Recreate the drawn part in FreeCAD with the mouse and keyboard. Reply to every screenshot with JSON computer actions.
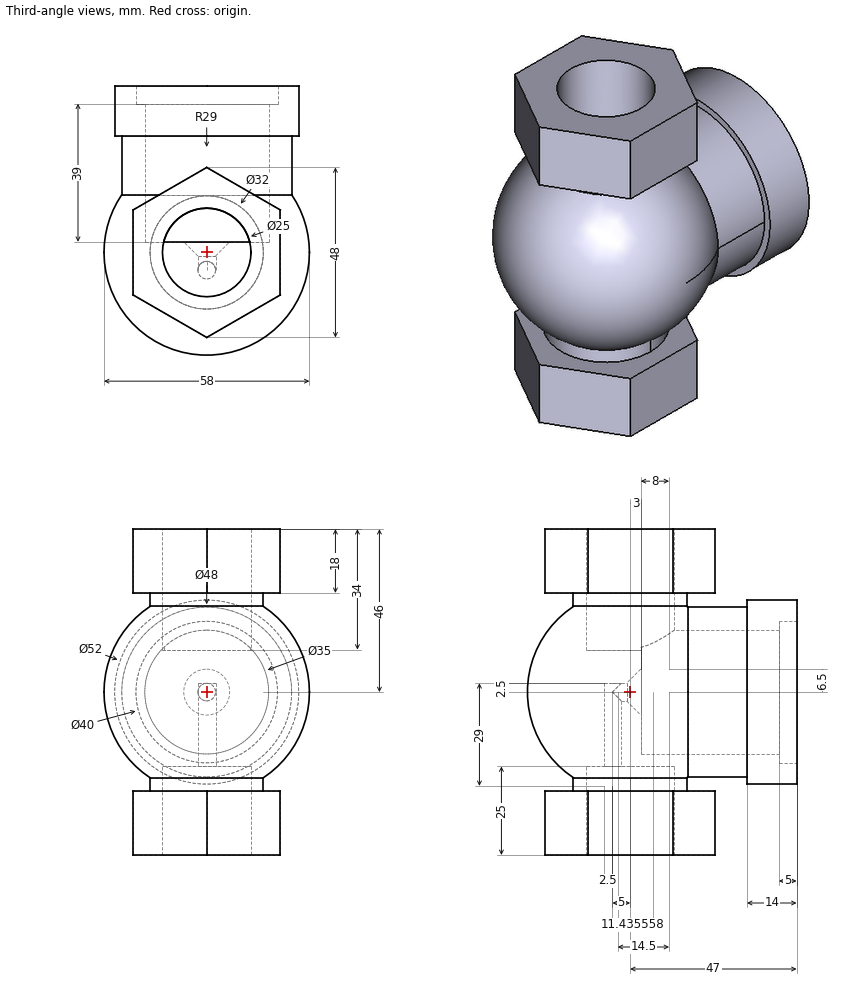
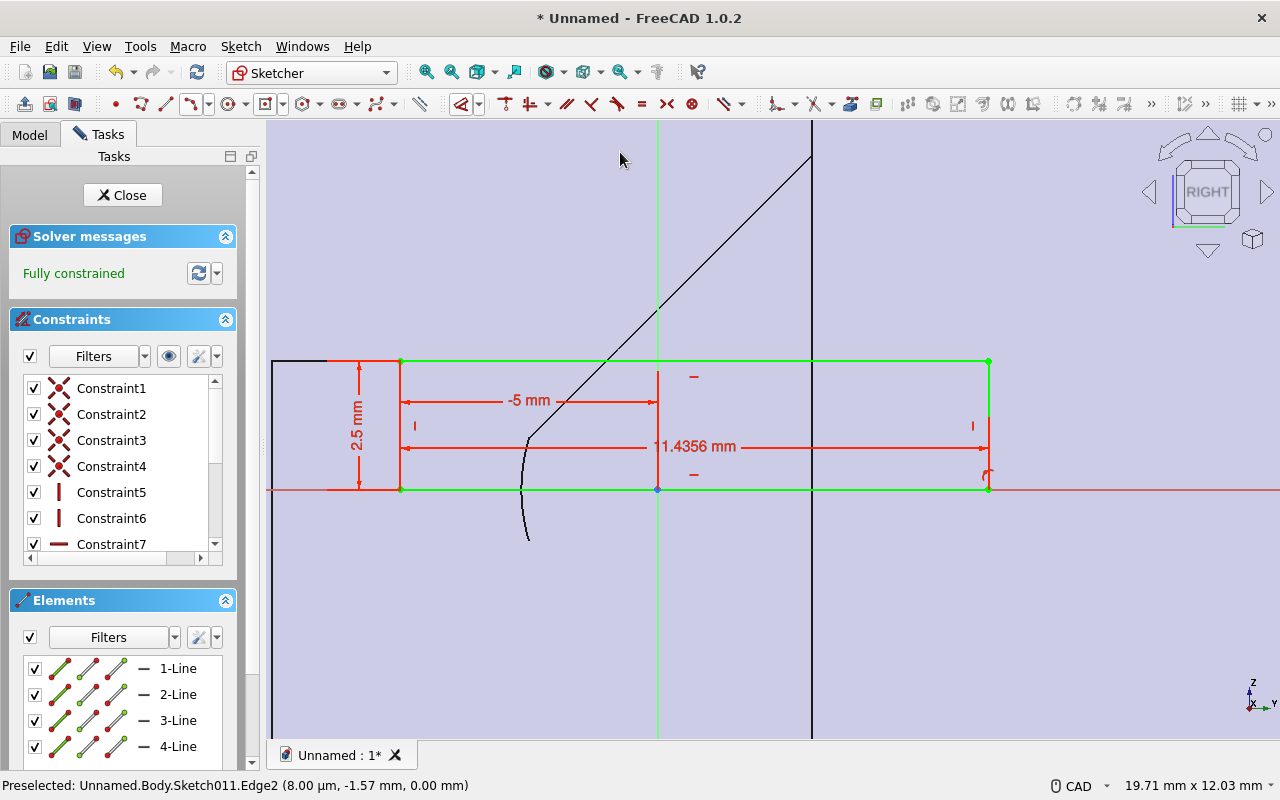
{"action": "left_click", "coordinate": [123, 195]}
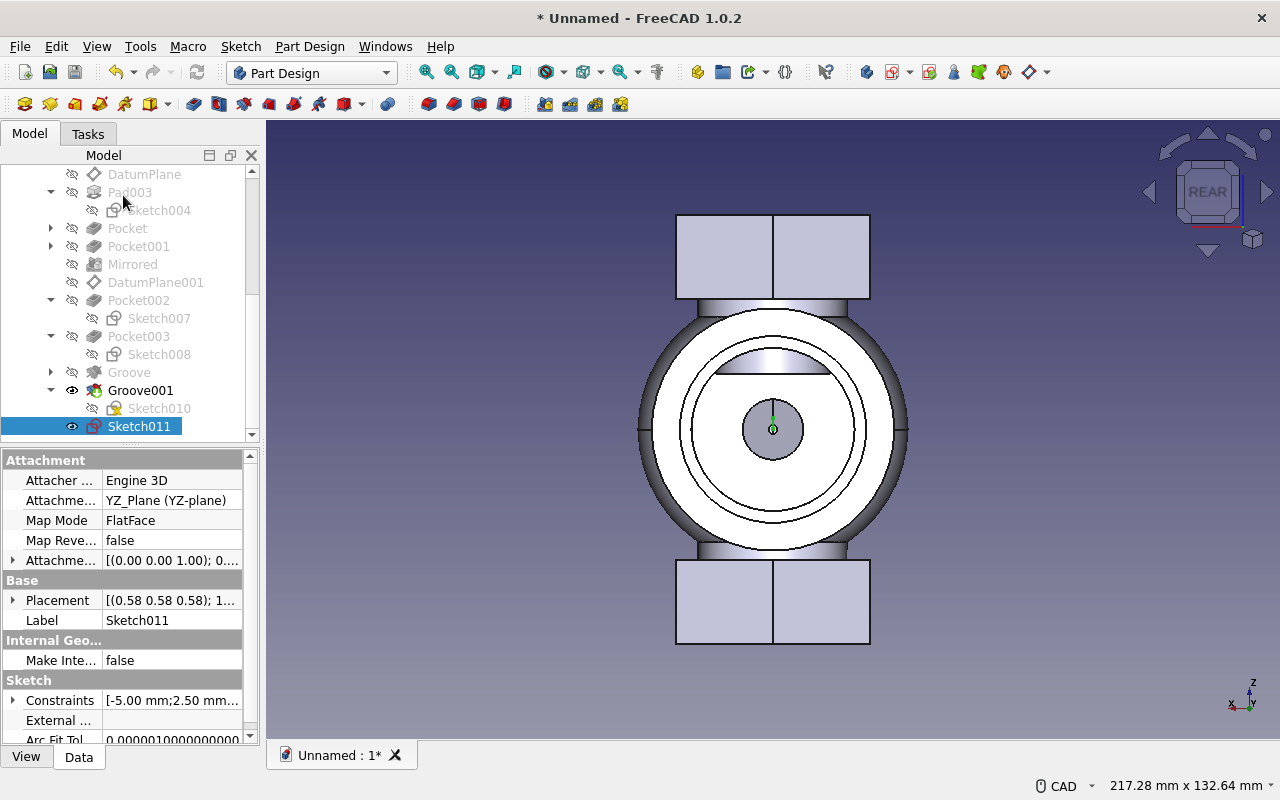
{"action": "left_click", "coordinate": [244, 104]}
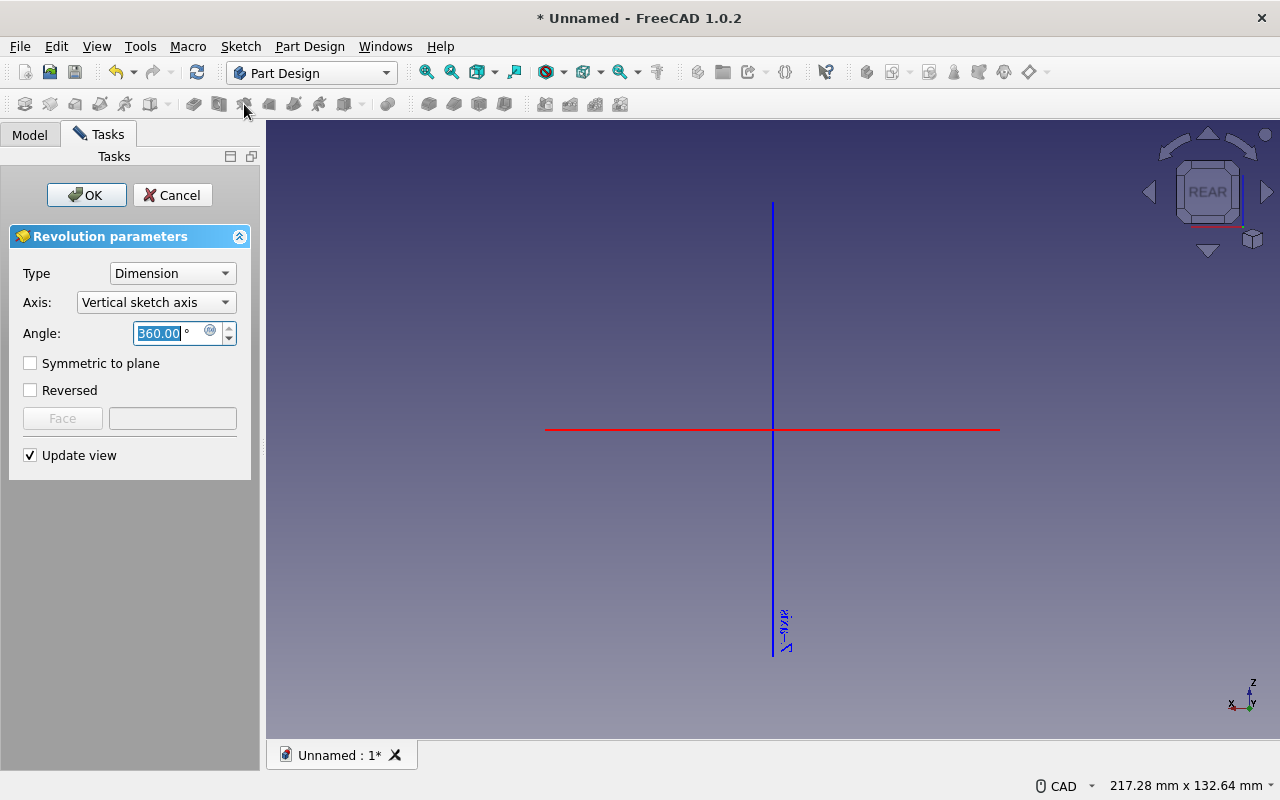
{"action": "left_click", "coordinate": [157, 302]}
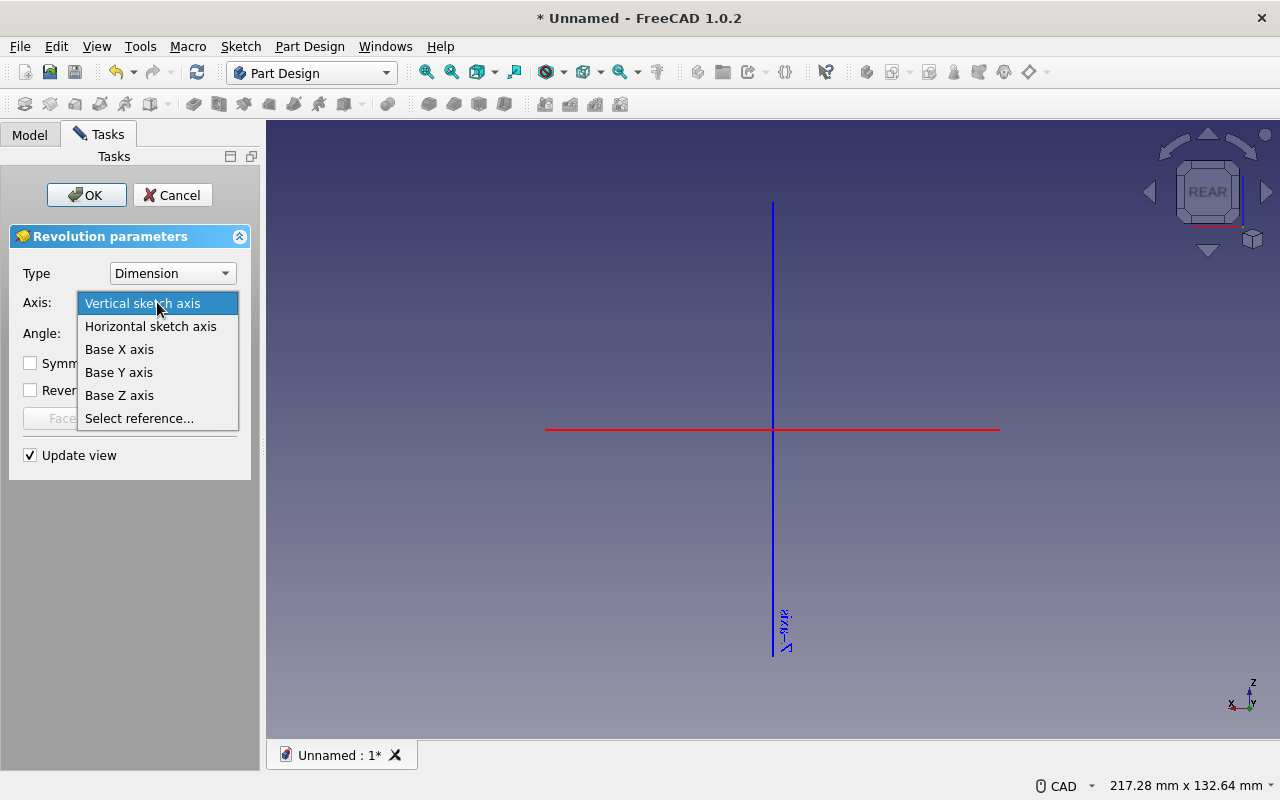
{"action": "left_click", "coordinate": [156, 326]}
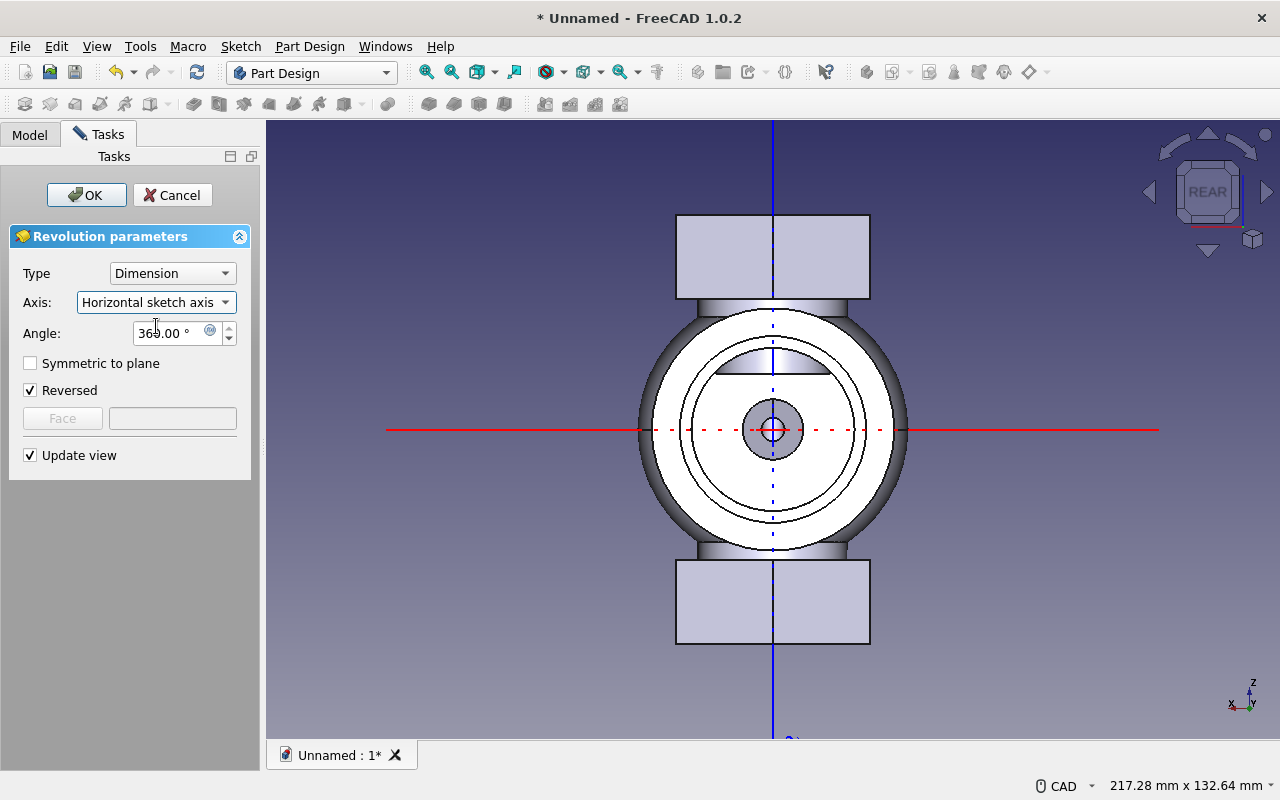
{"action": "left_click", "coordinate": [87, 195]}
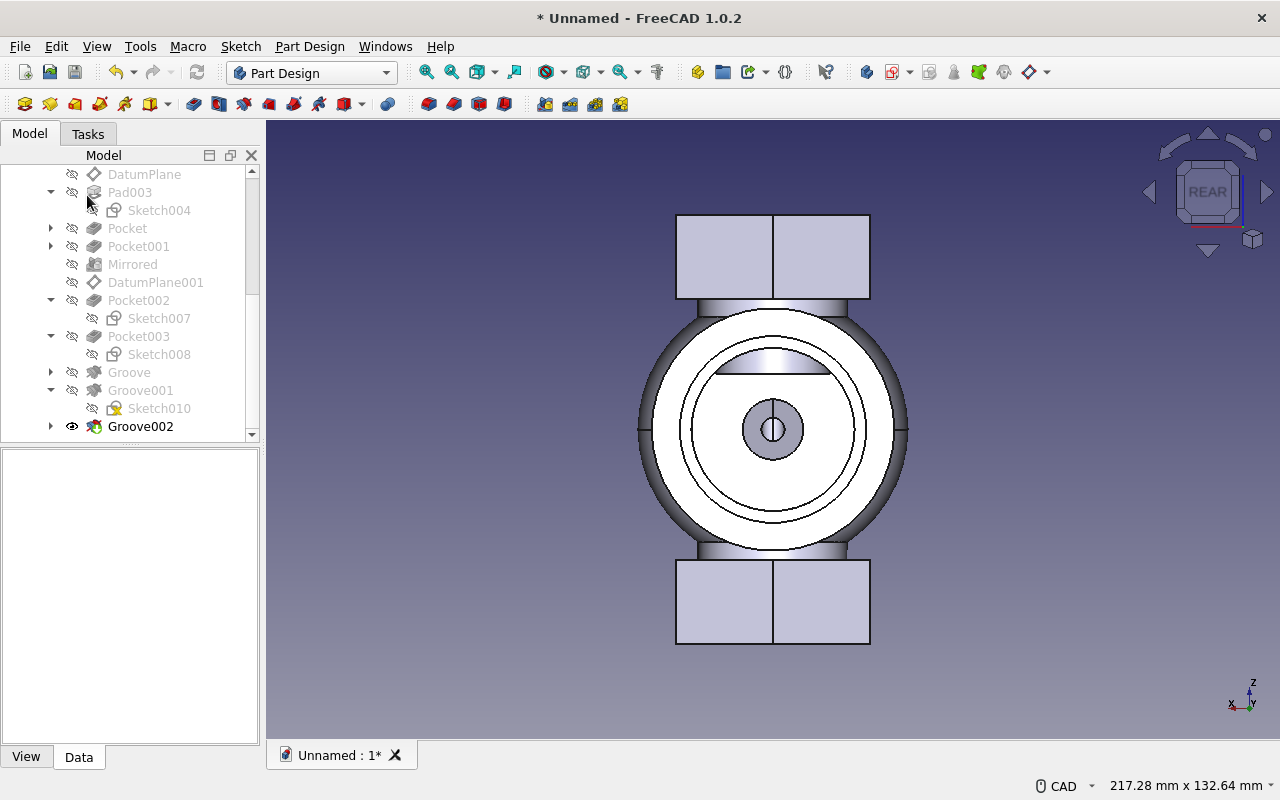
{"action": "key", "text": "0"}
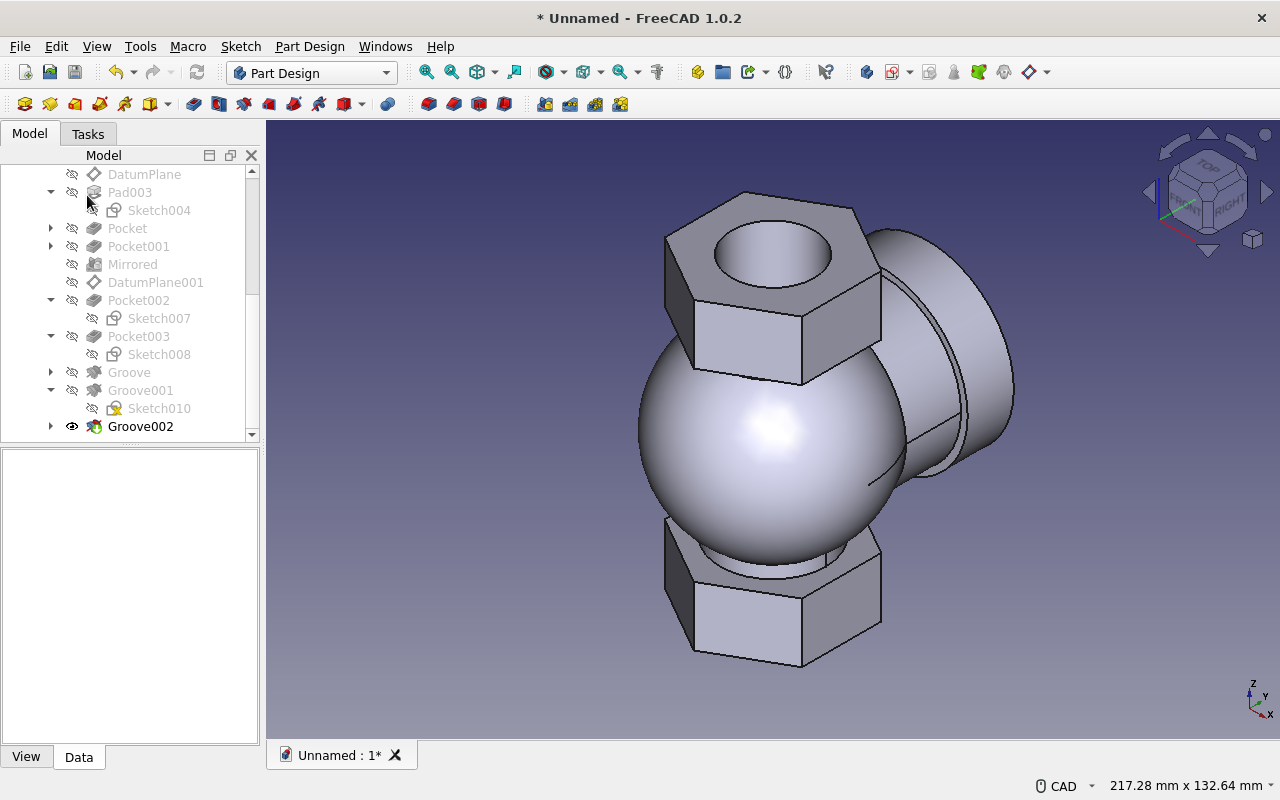
{"action": "left_click", "coordinate": [427, 72]}